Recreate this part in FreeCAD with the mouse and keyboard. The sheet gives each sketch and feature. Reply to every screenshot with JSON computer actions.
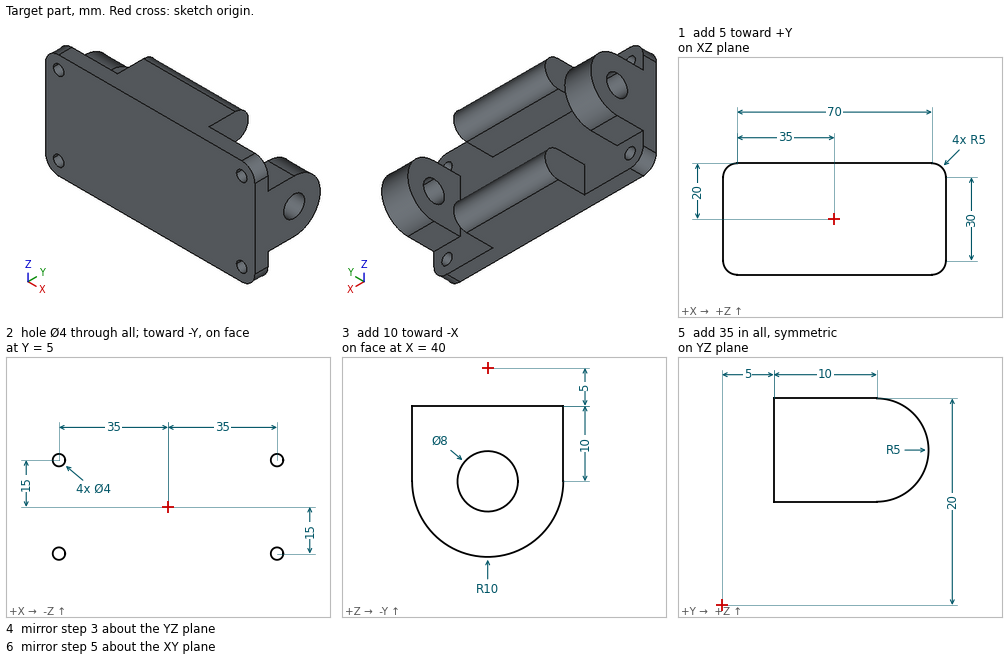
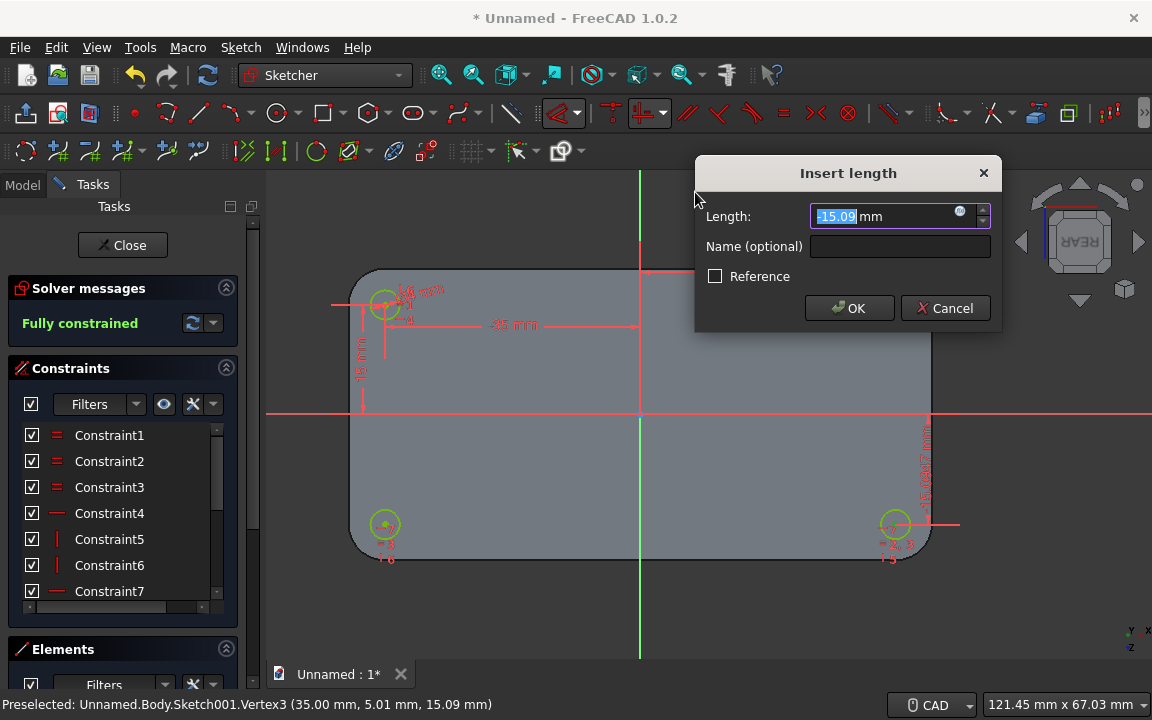
{"action": "type", "text": "-15"}
{"action": "key", "text": "Return"}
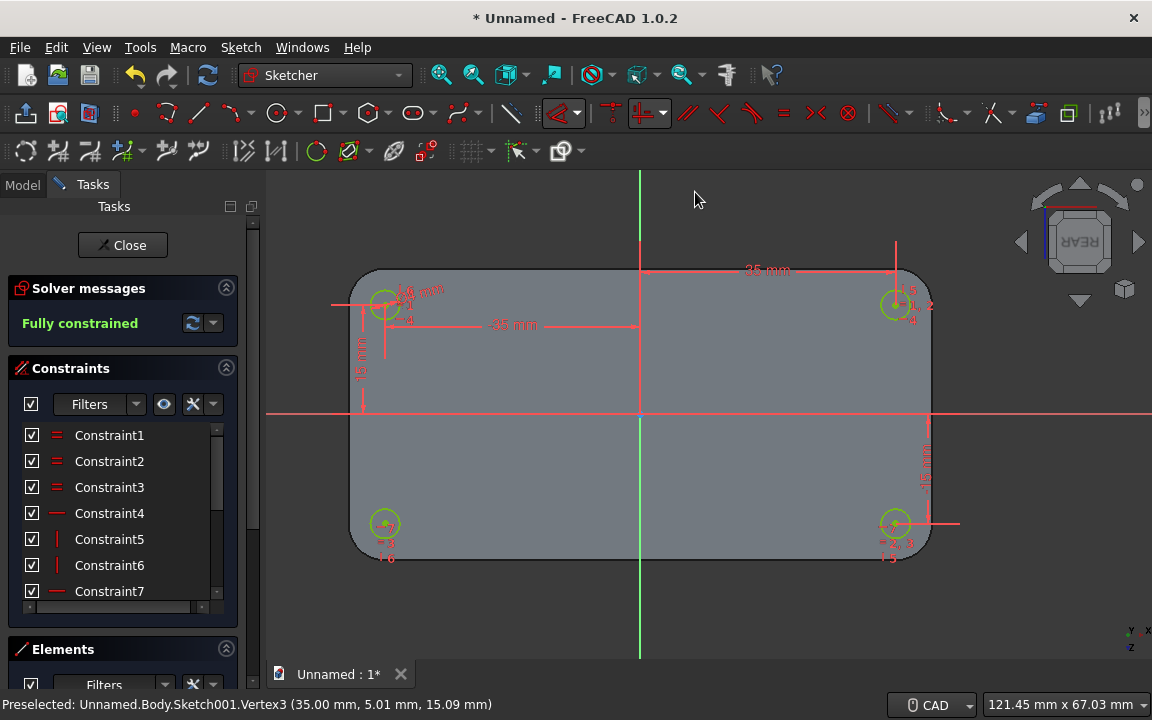
{"action": "left_click", "coordinate": [123, 245]}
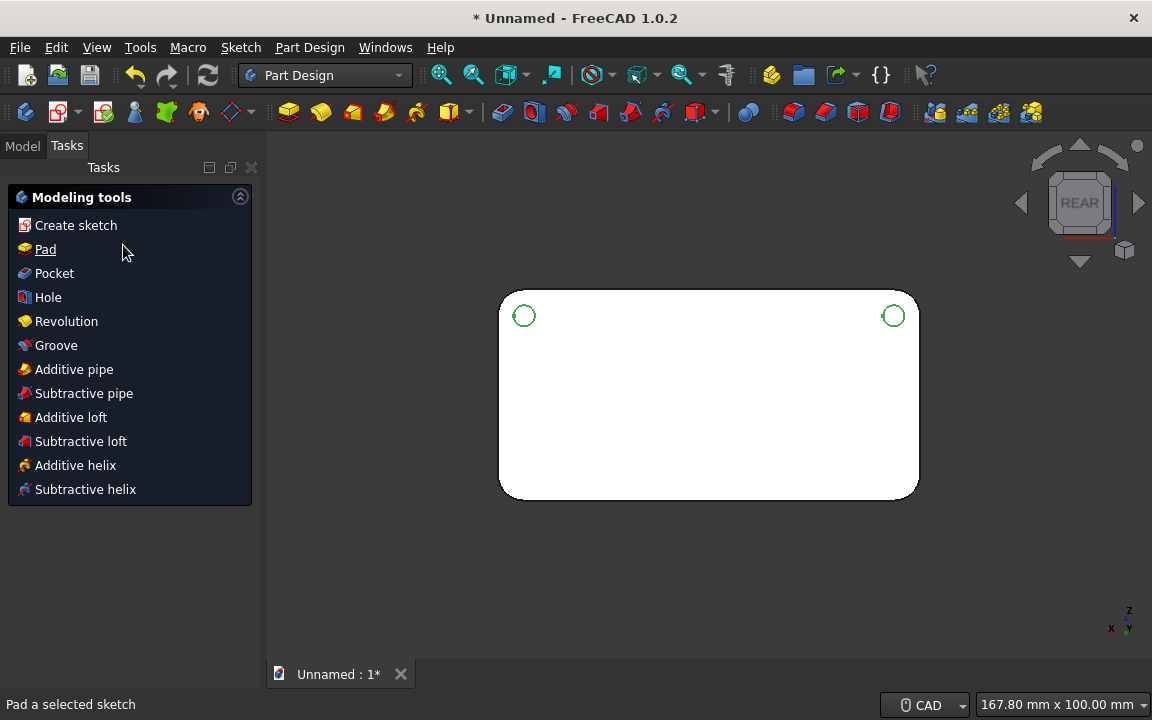
{"action": "left_click", "coordinate": [536, 112]}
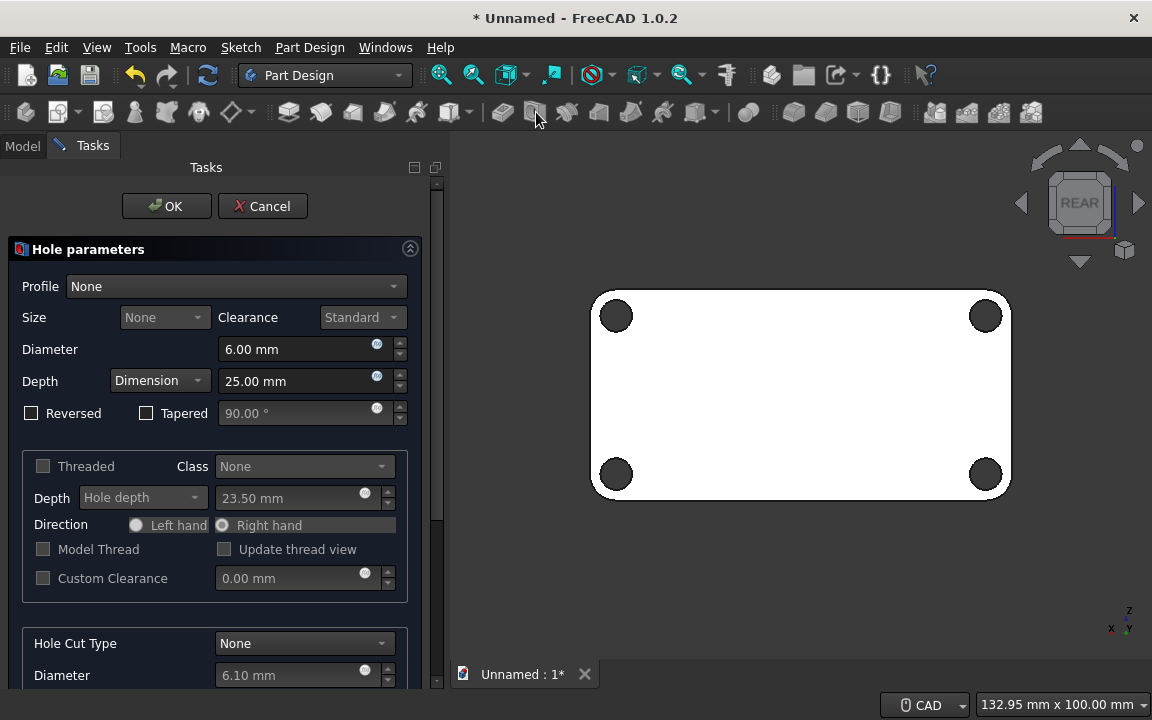
{"action": "triple_click", "coordinate": [305, 349]}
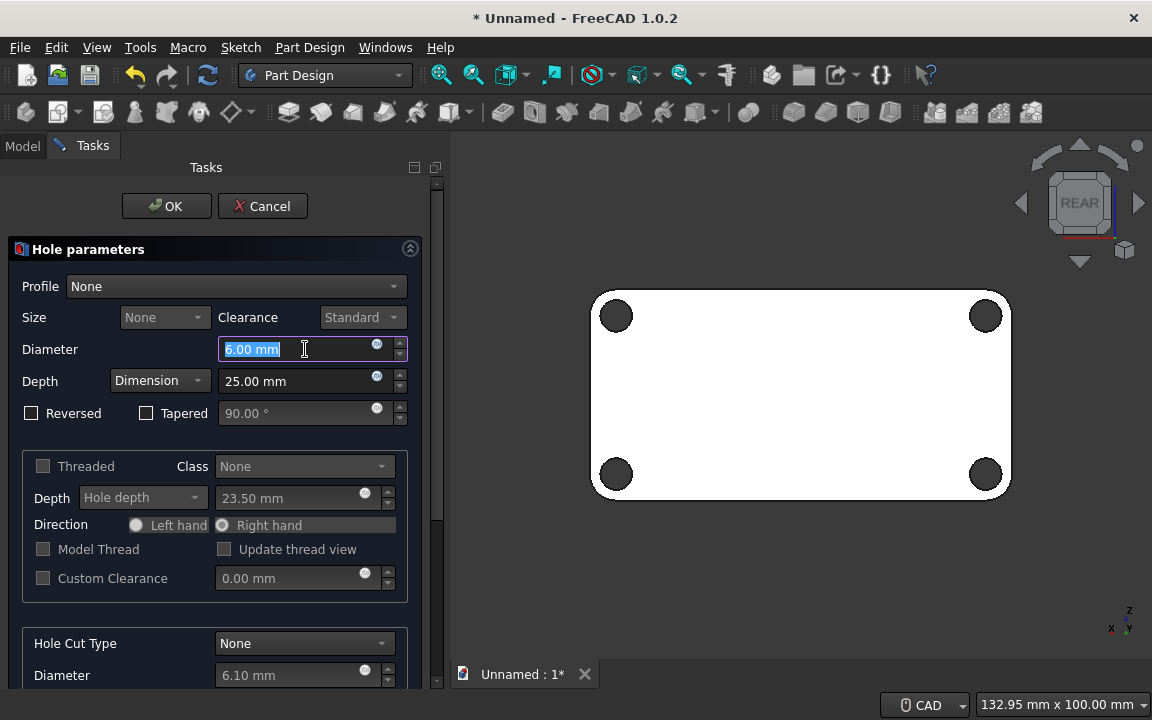
{"action": "type", "text": "4"}
{"action": "key", "text": "Tab"}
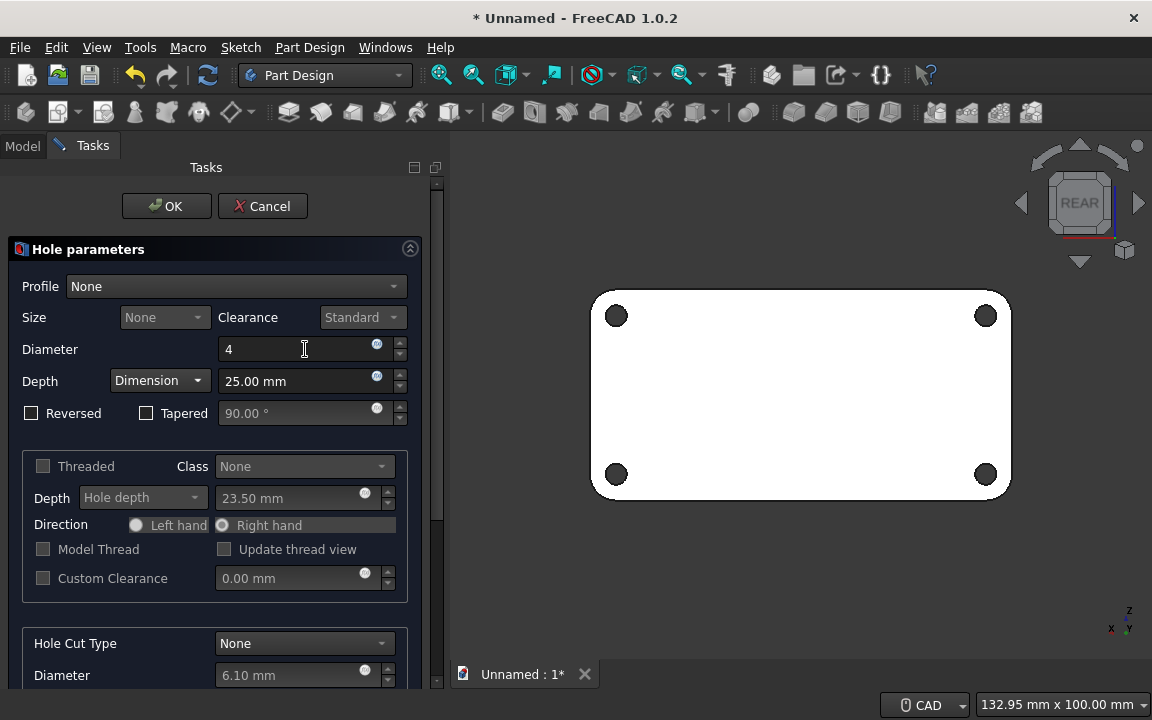
{"action": "left_click", "coordinate": [161, 380]}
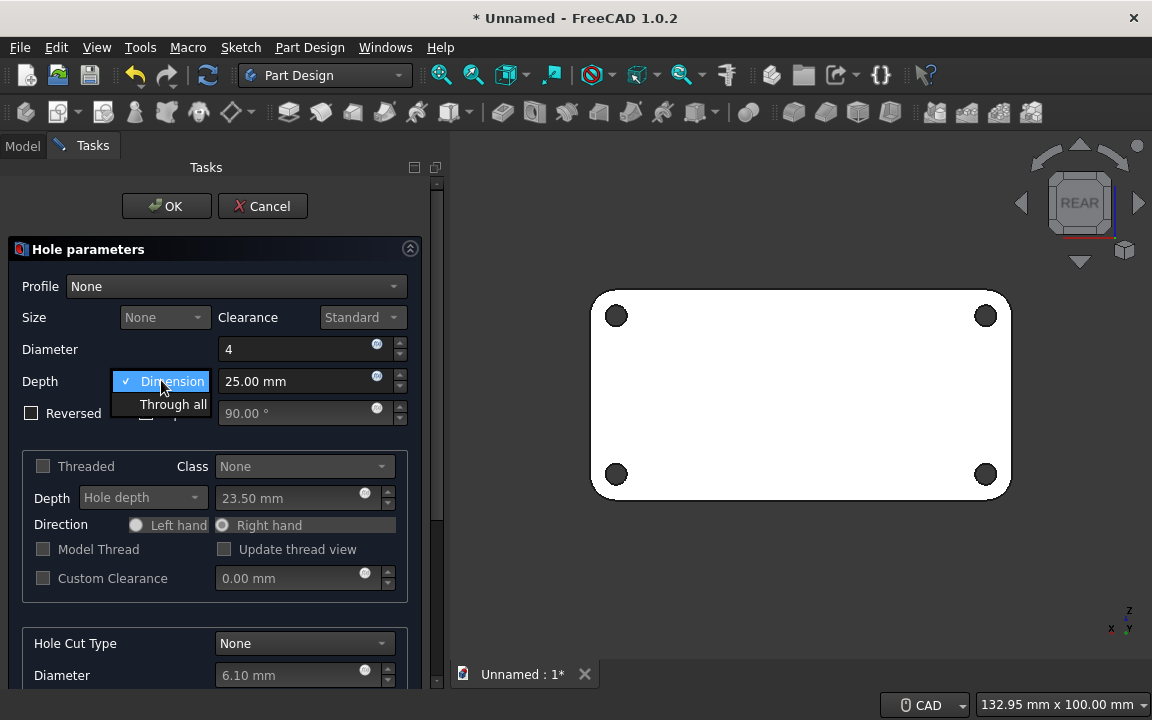
{"action": "left_click", "coordinate": [160, 404]}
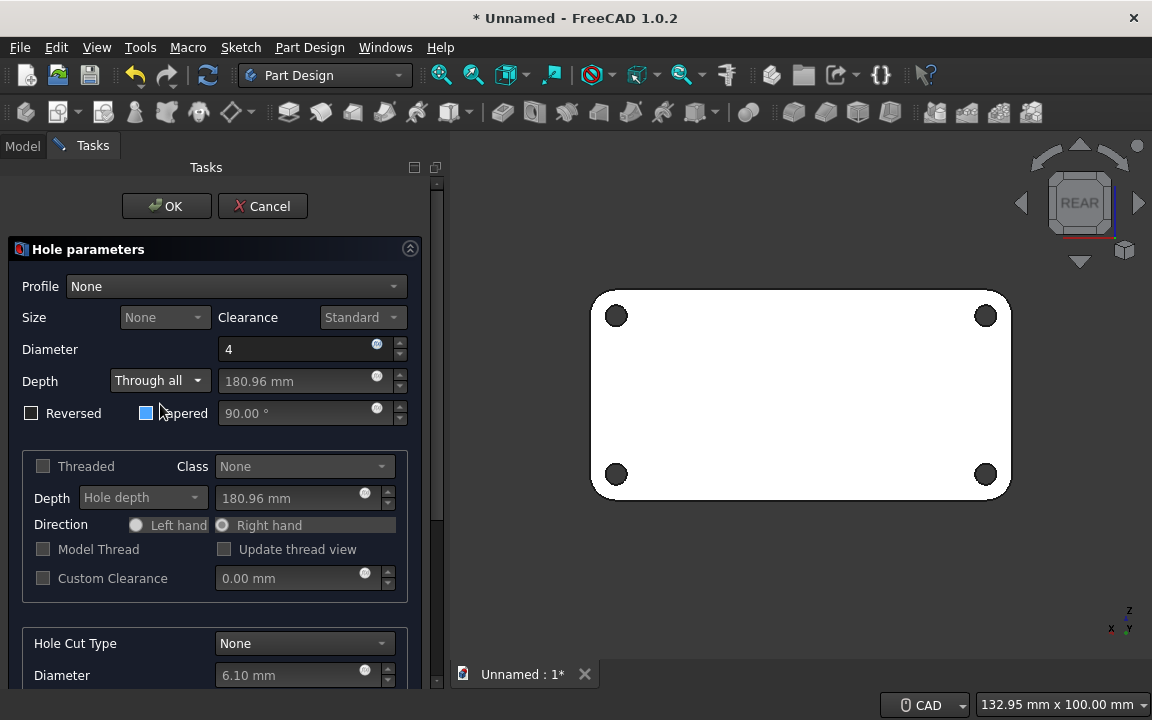
{"action": "left_click", "coordinate": [167, 206]}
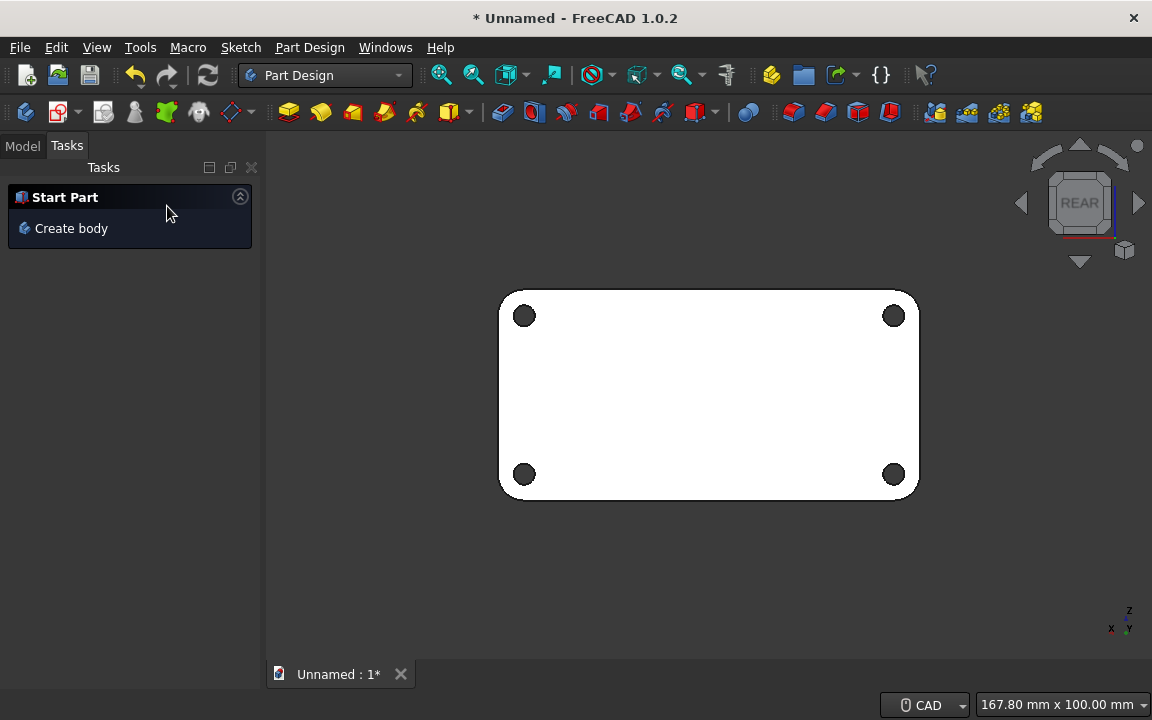
{"action": "key", "text": "0"}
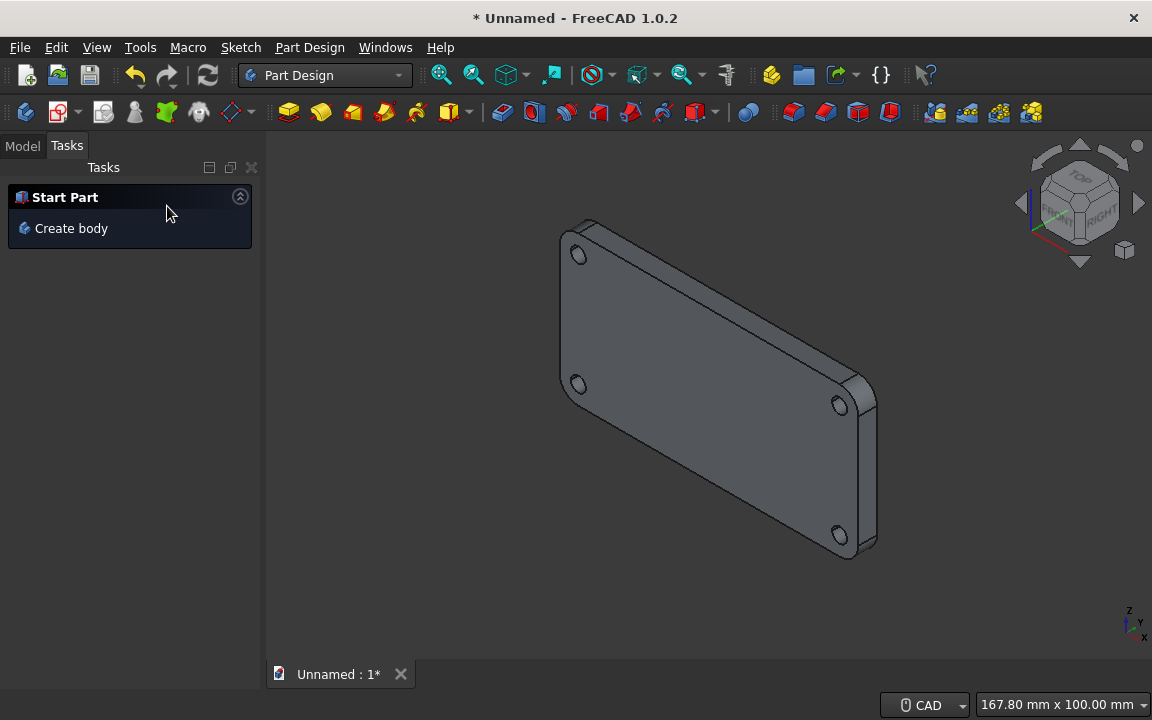
{"action": "left_click", "coordinate": [868, 475]}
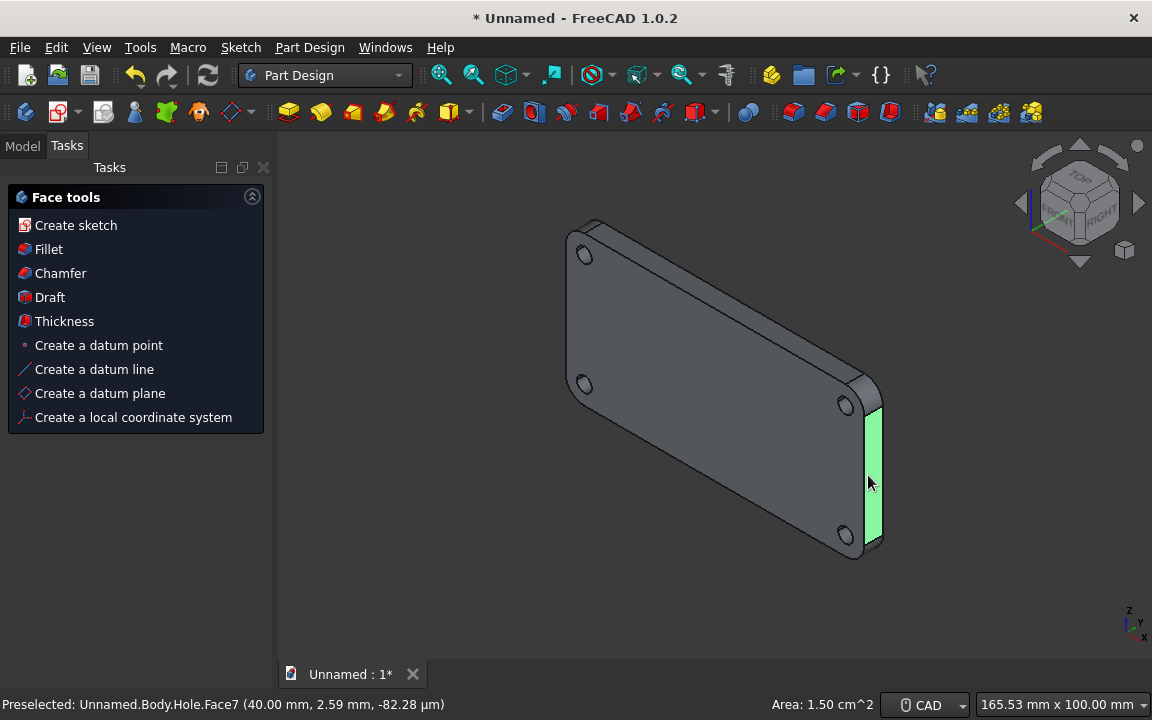
{"action": "left_click", "coordinate": [58, 112]}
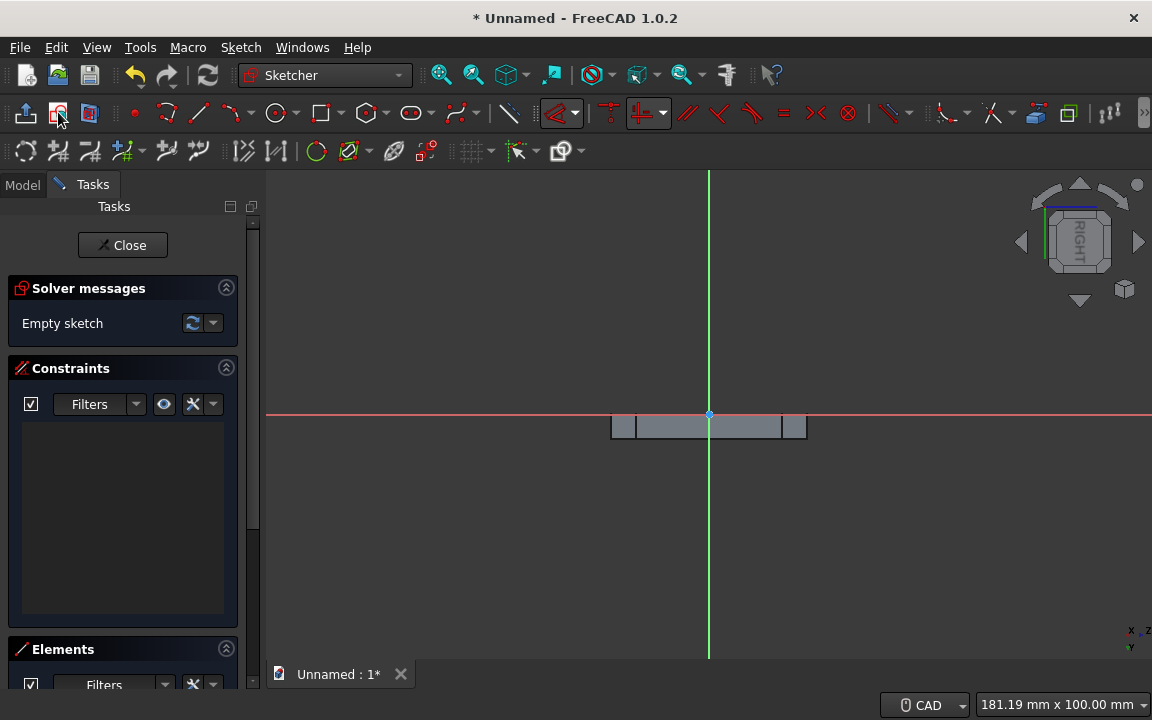
{"action": "scroll", "coordinate": [749, 511], "scroll_direction": "up", "scroll_amount": 5}